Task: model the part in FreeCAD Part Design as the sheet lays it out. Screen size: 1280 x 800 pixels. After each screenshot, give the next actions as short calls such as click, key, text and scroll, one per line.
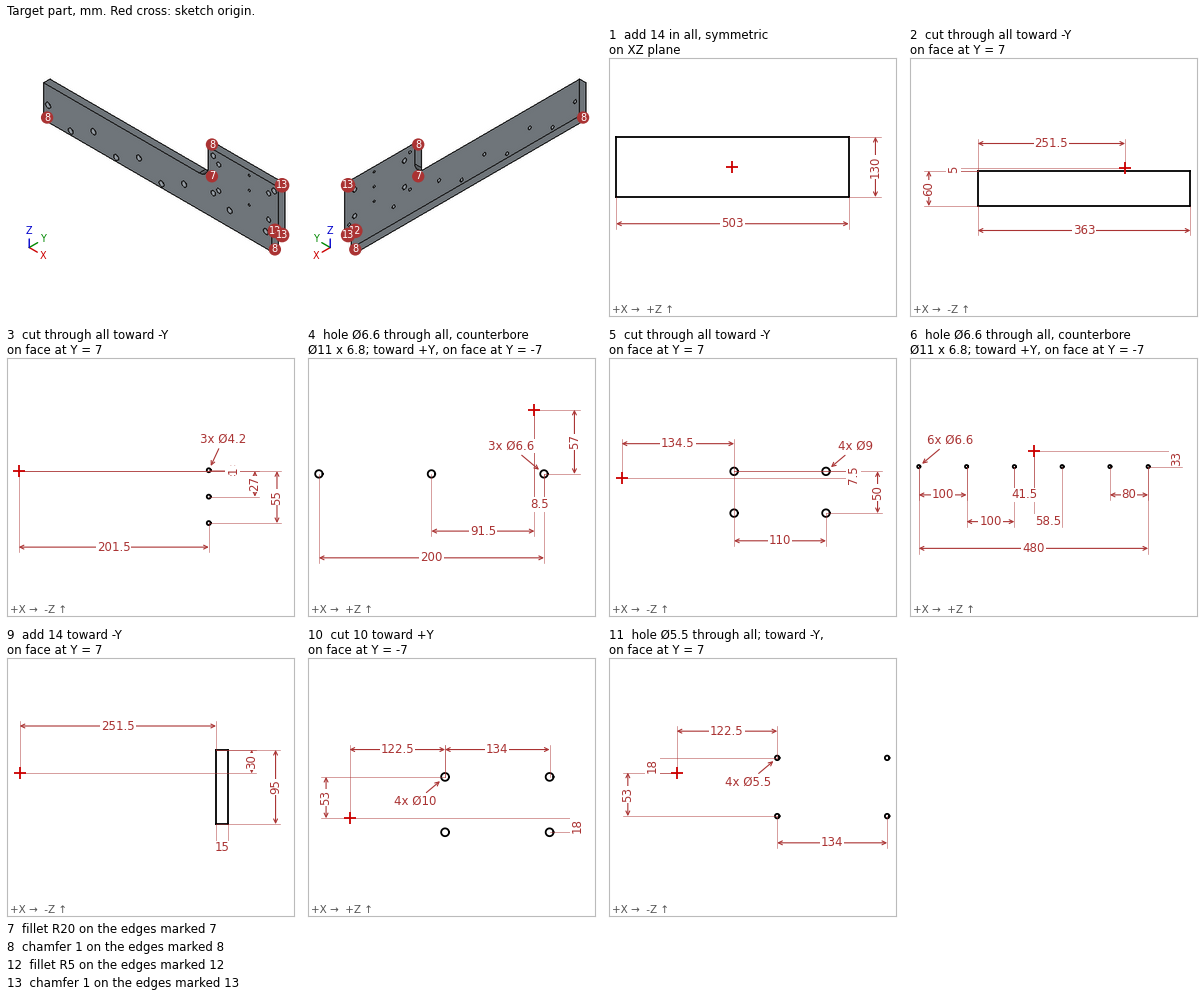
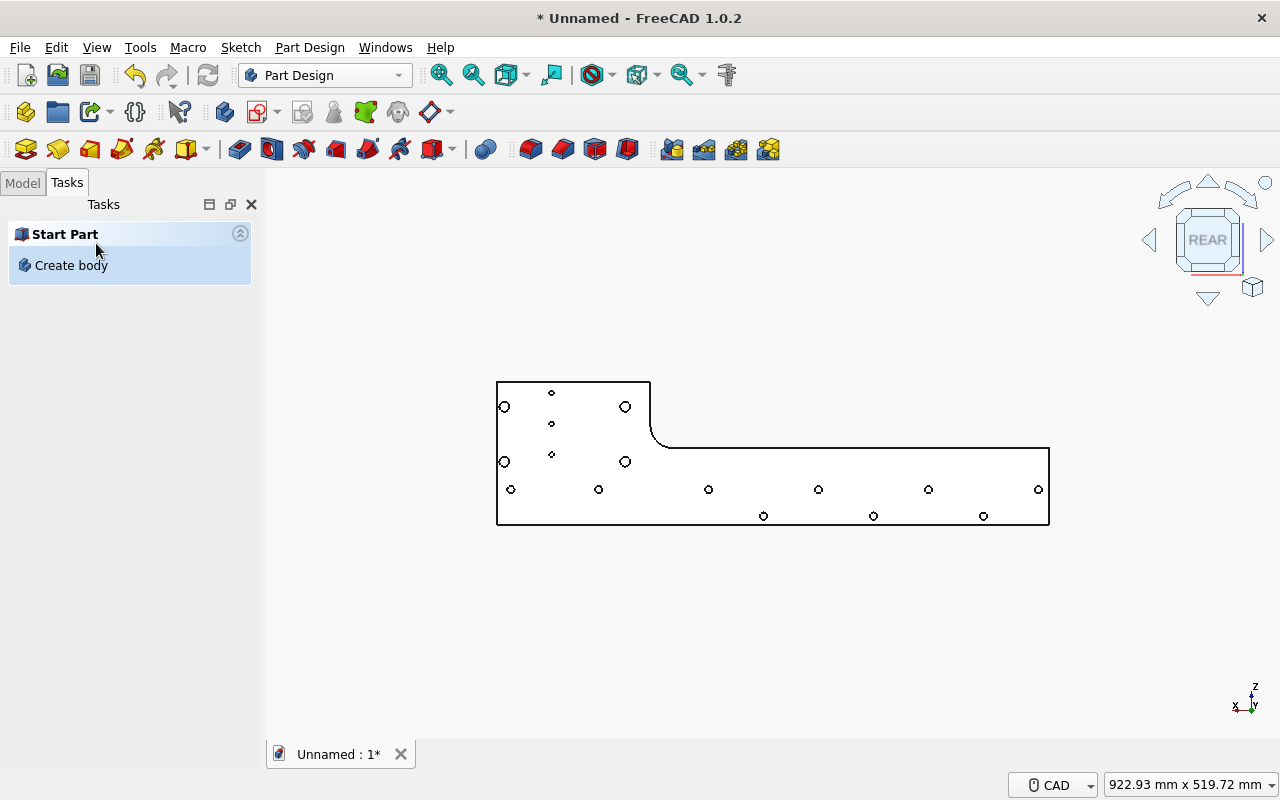
click(852, 493)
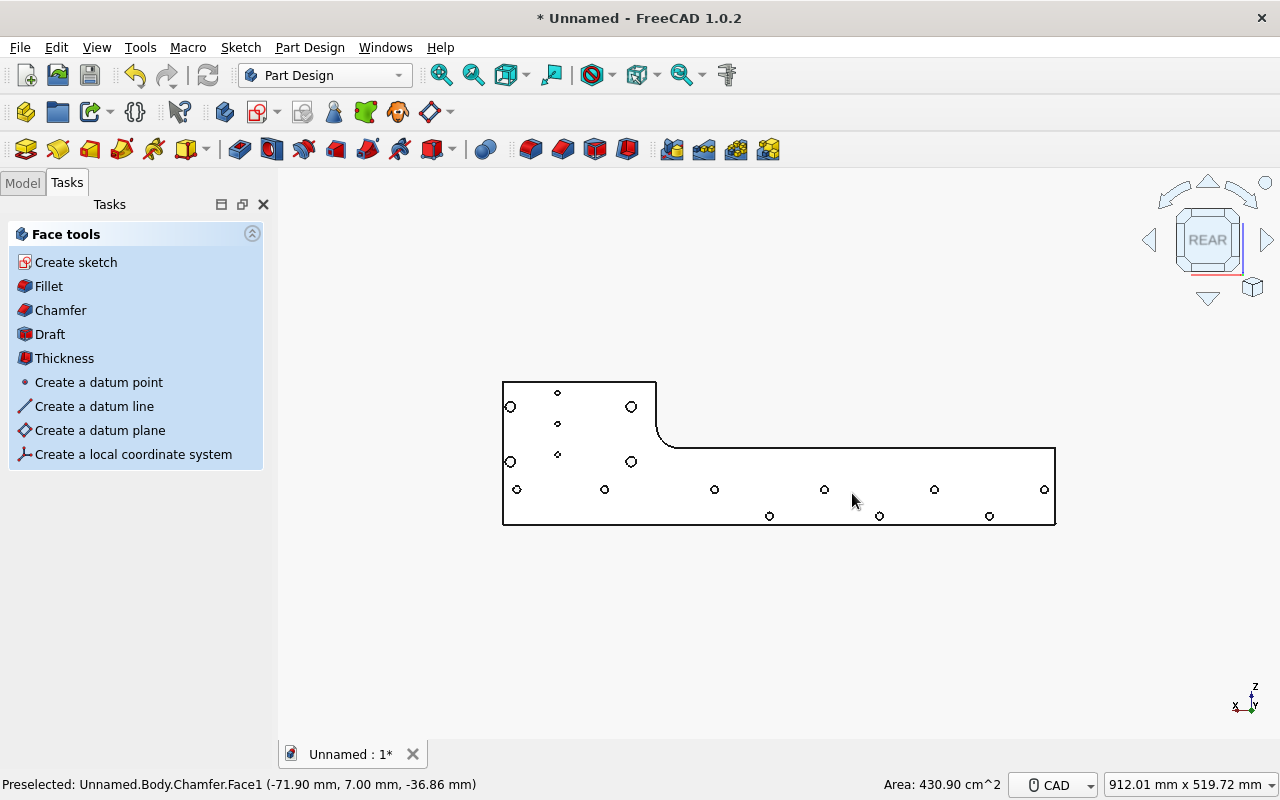
click(258, 112)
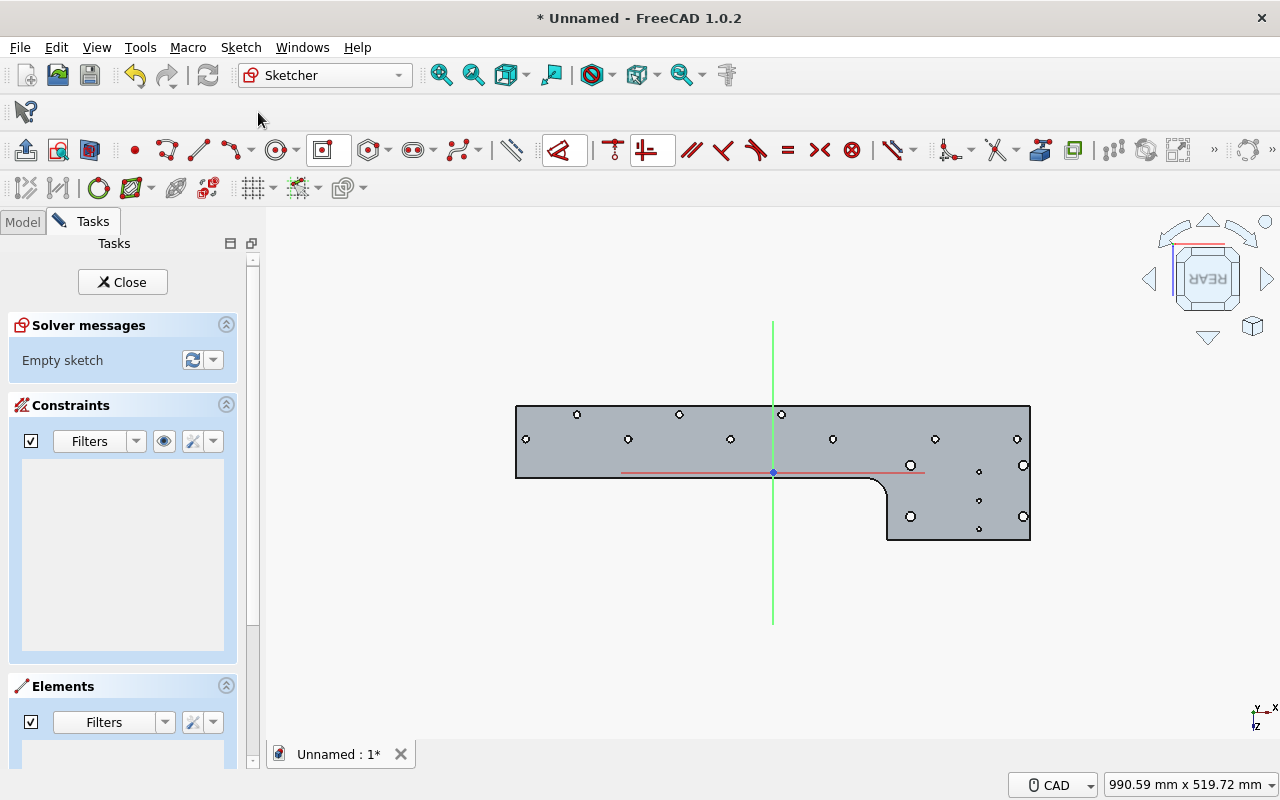
scroll(1115, 499, up, 6)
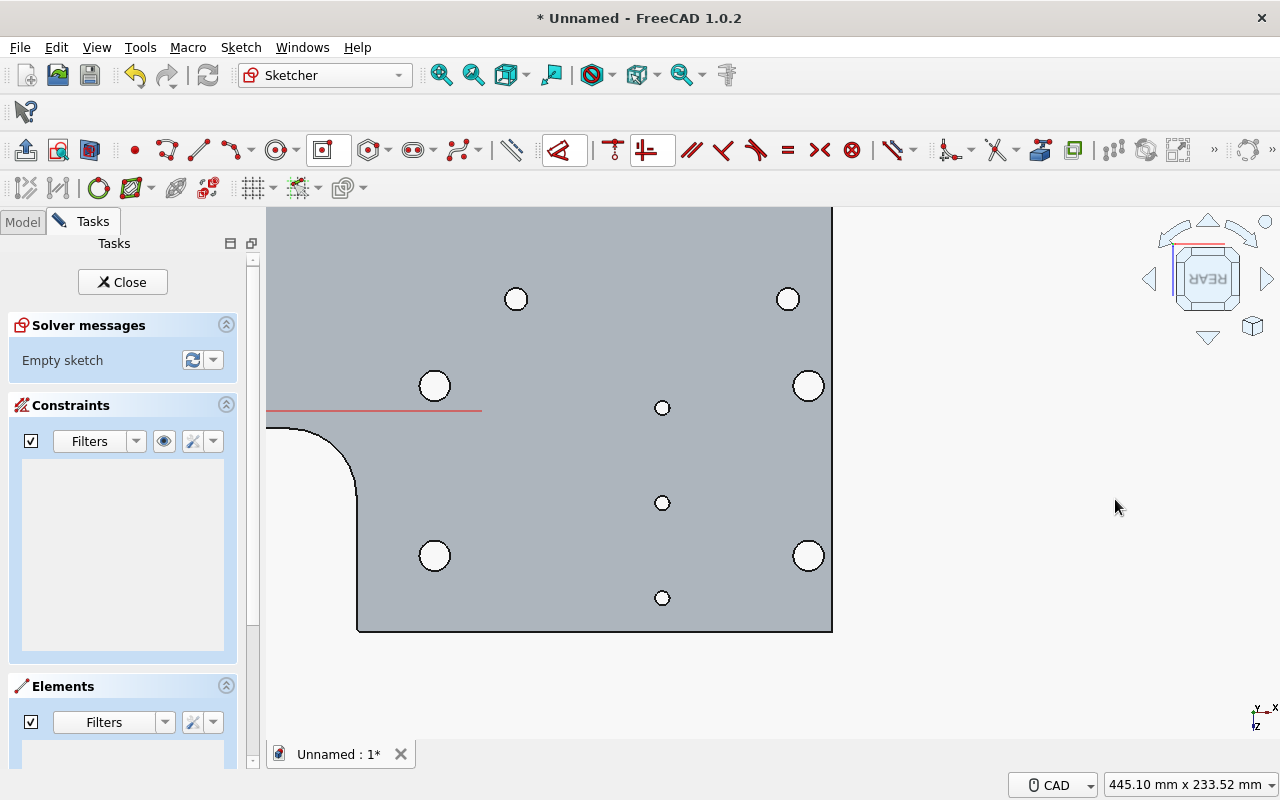
click(346, 150)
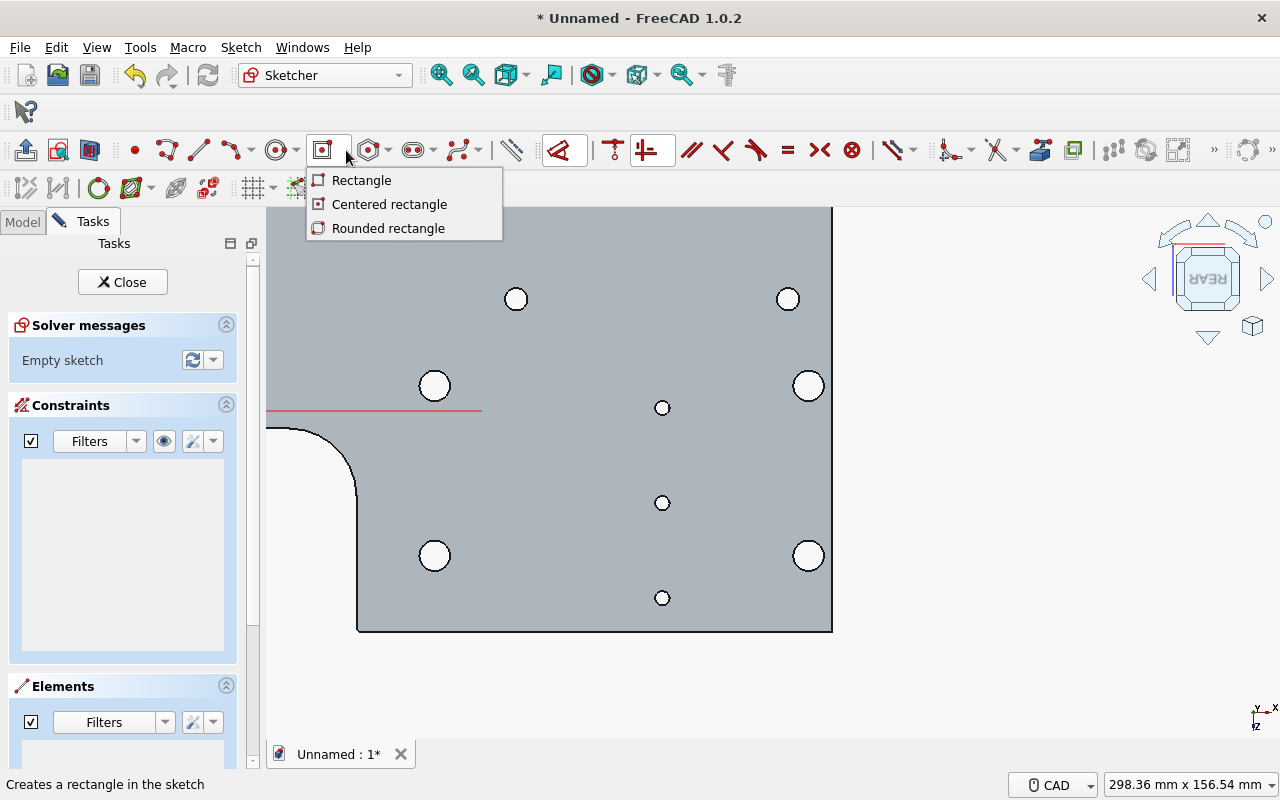
click(404, 180)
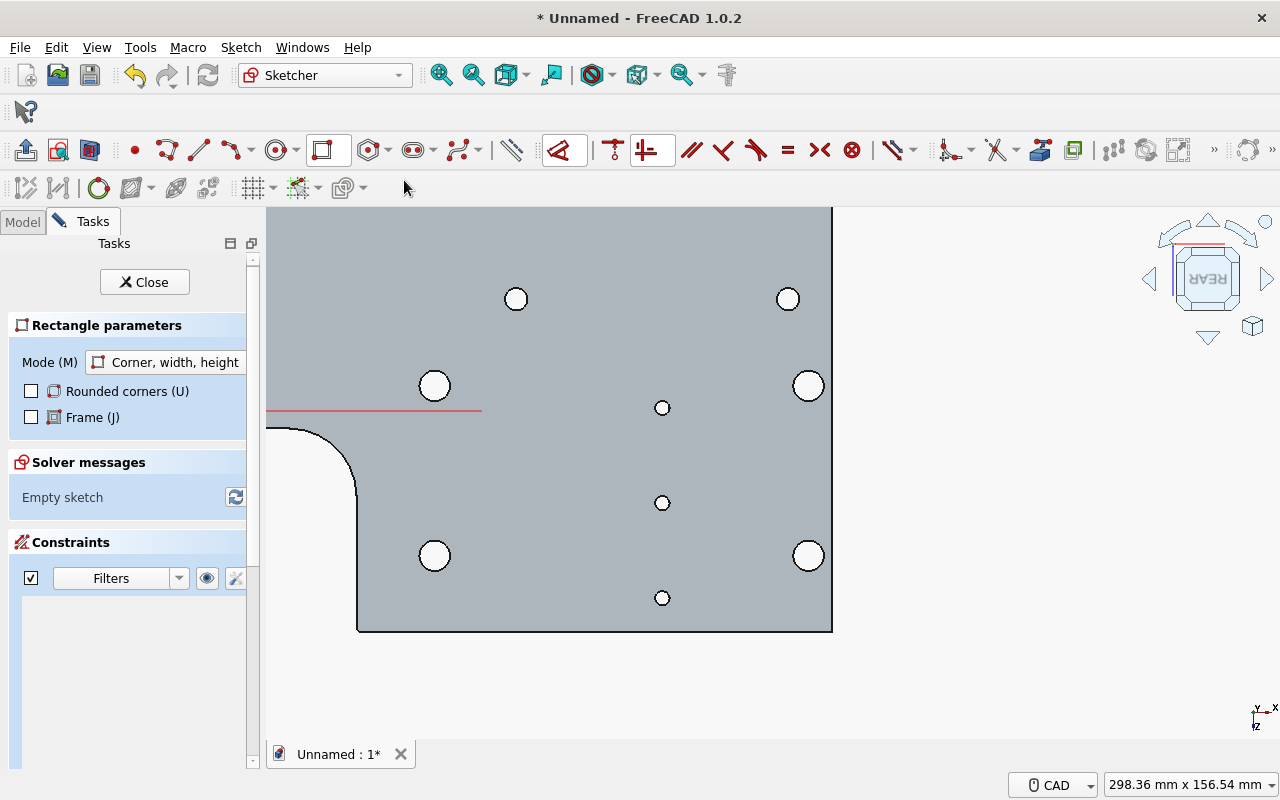
click(832, 309)
click(883, 632)
key(Escape)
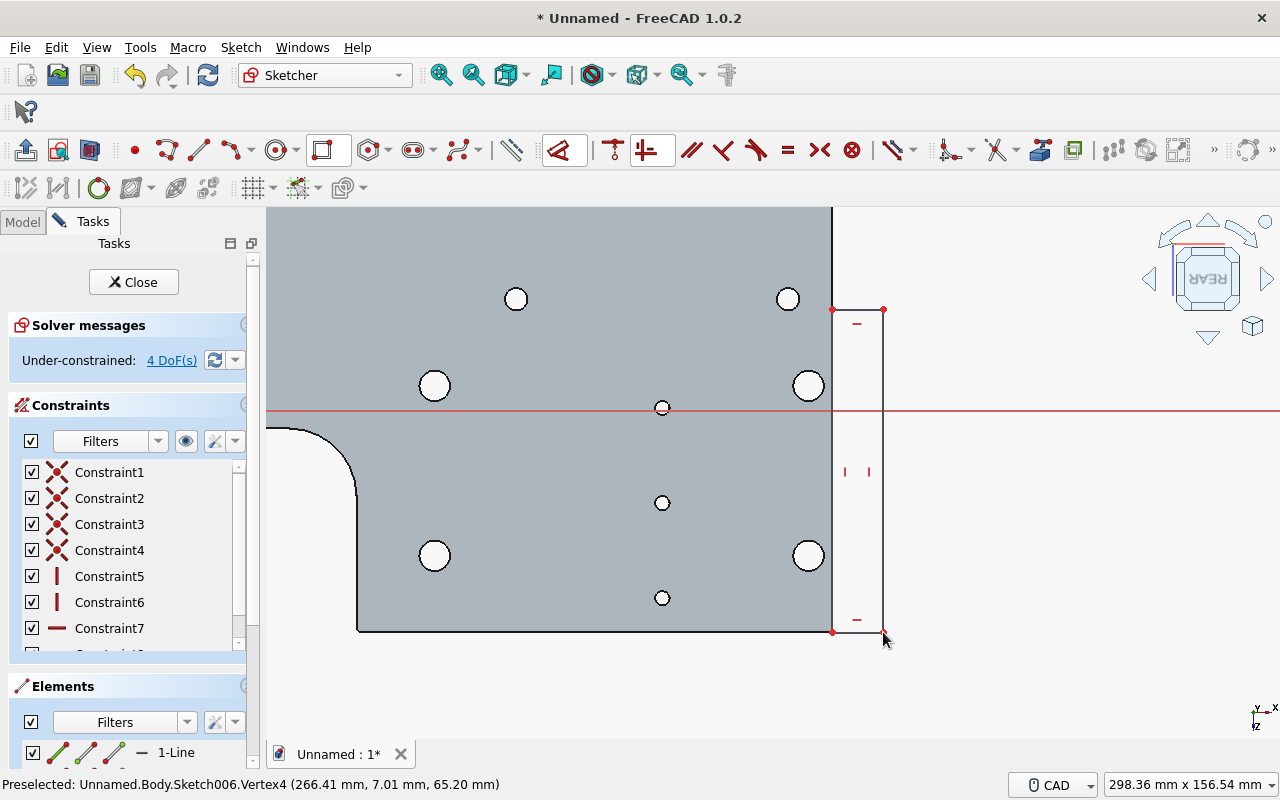
click(832, 536)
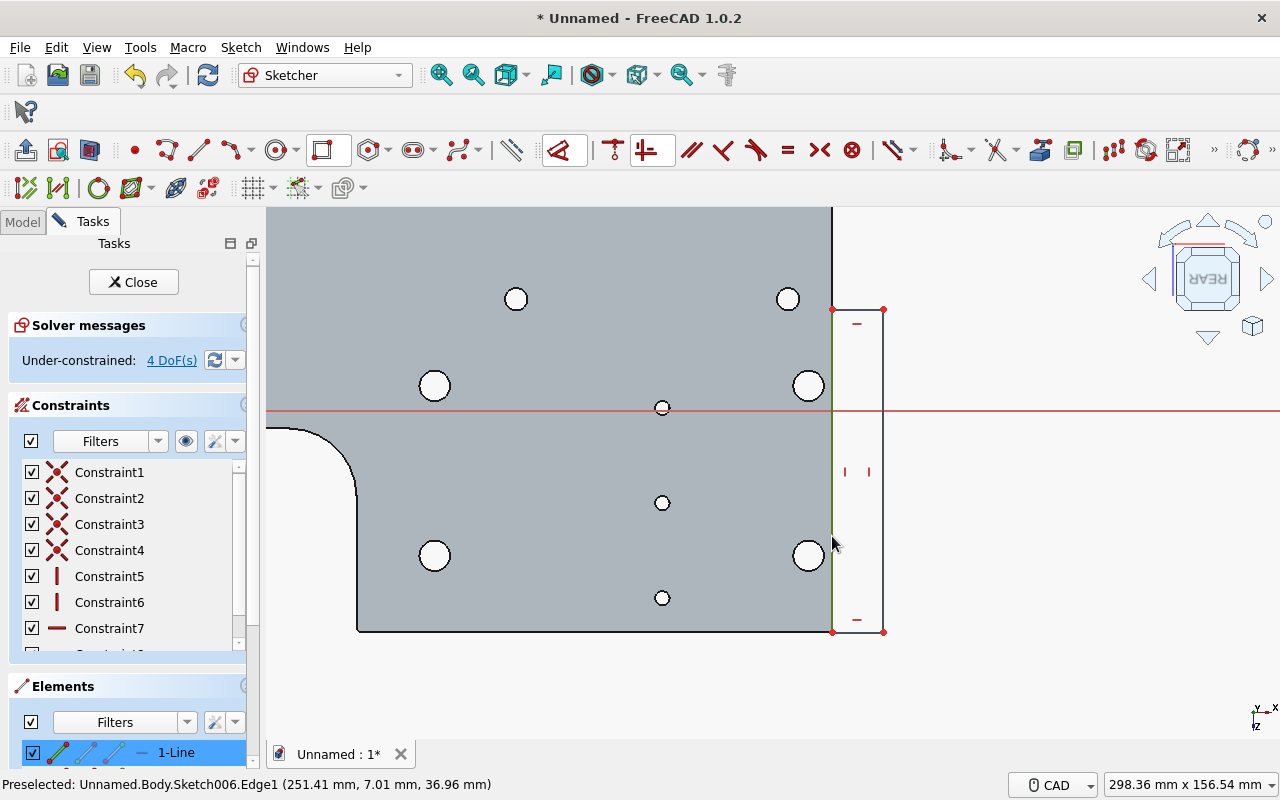
key(i)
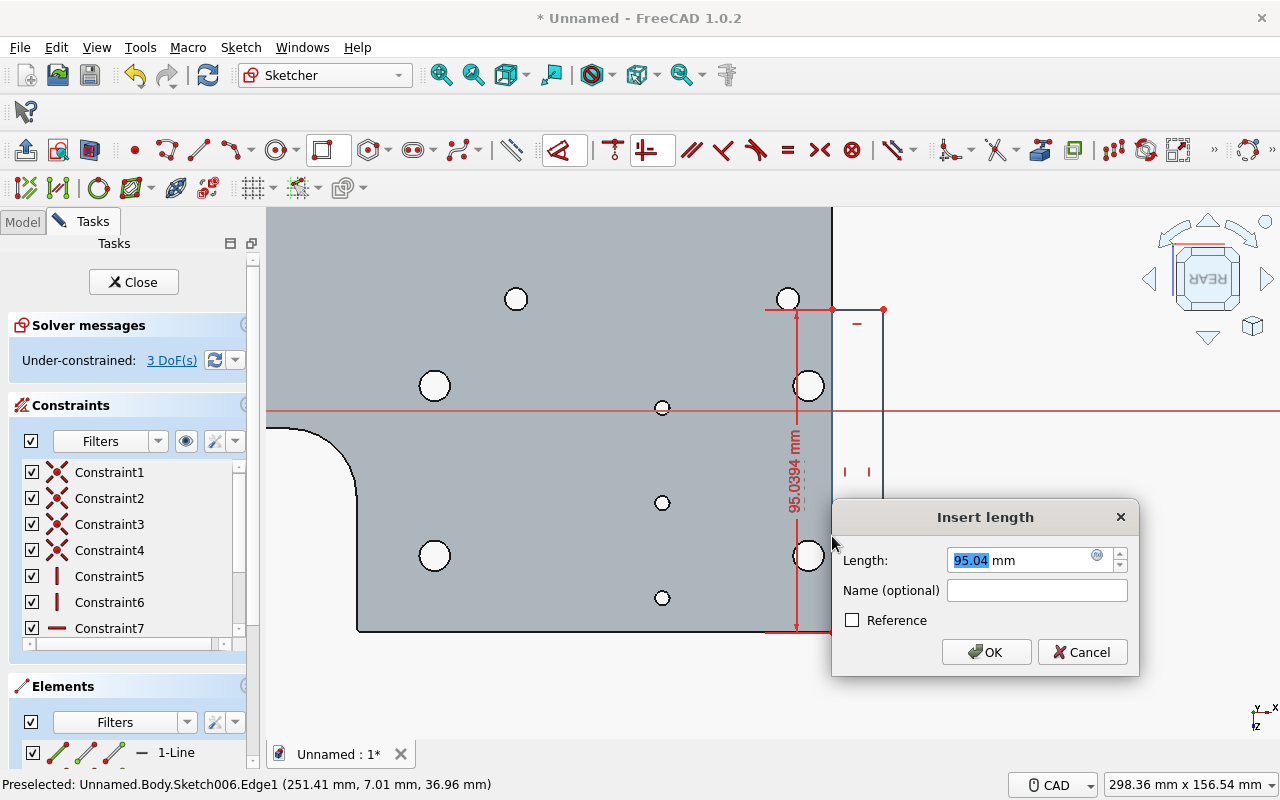
text(95)
key(Return)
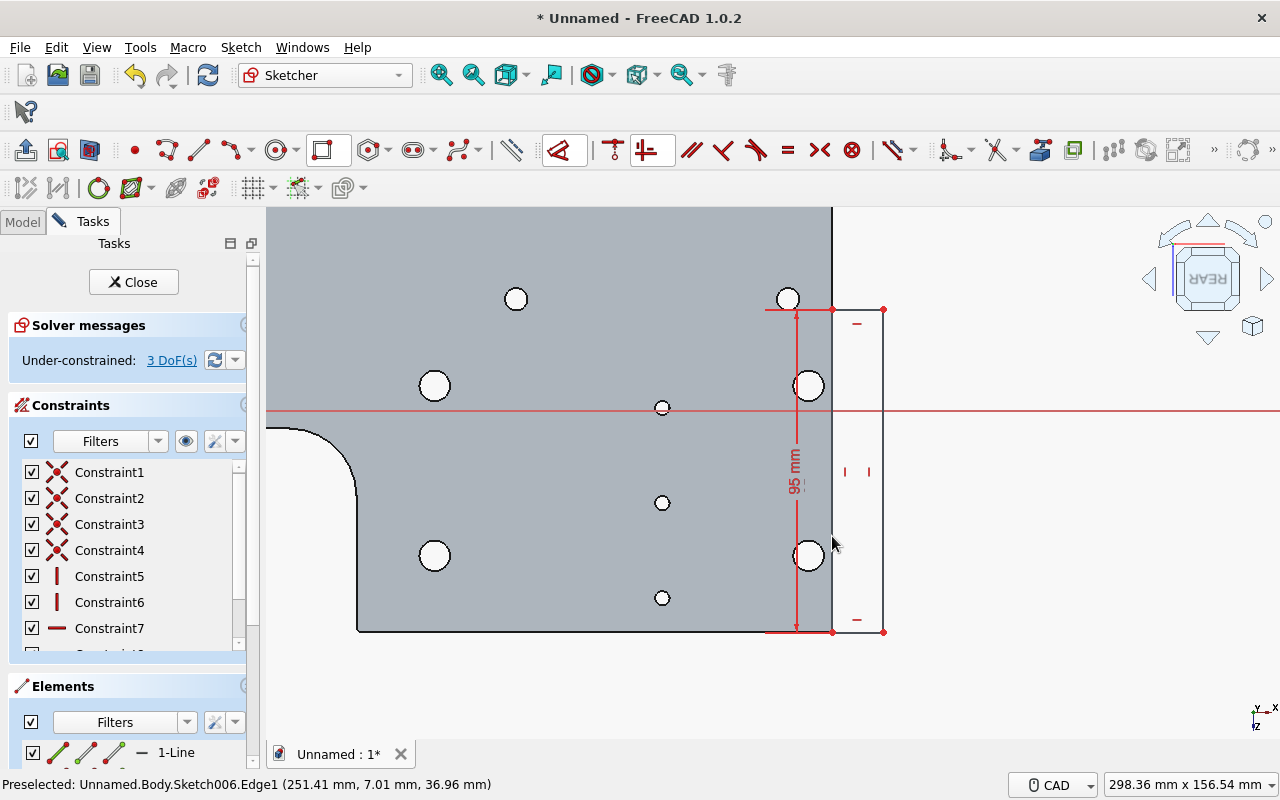
click(847, 633)